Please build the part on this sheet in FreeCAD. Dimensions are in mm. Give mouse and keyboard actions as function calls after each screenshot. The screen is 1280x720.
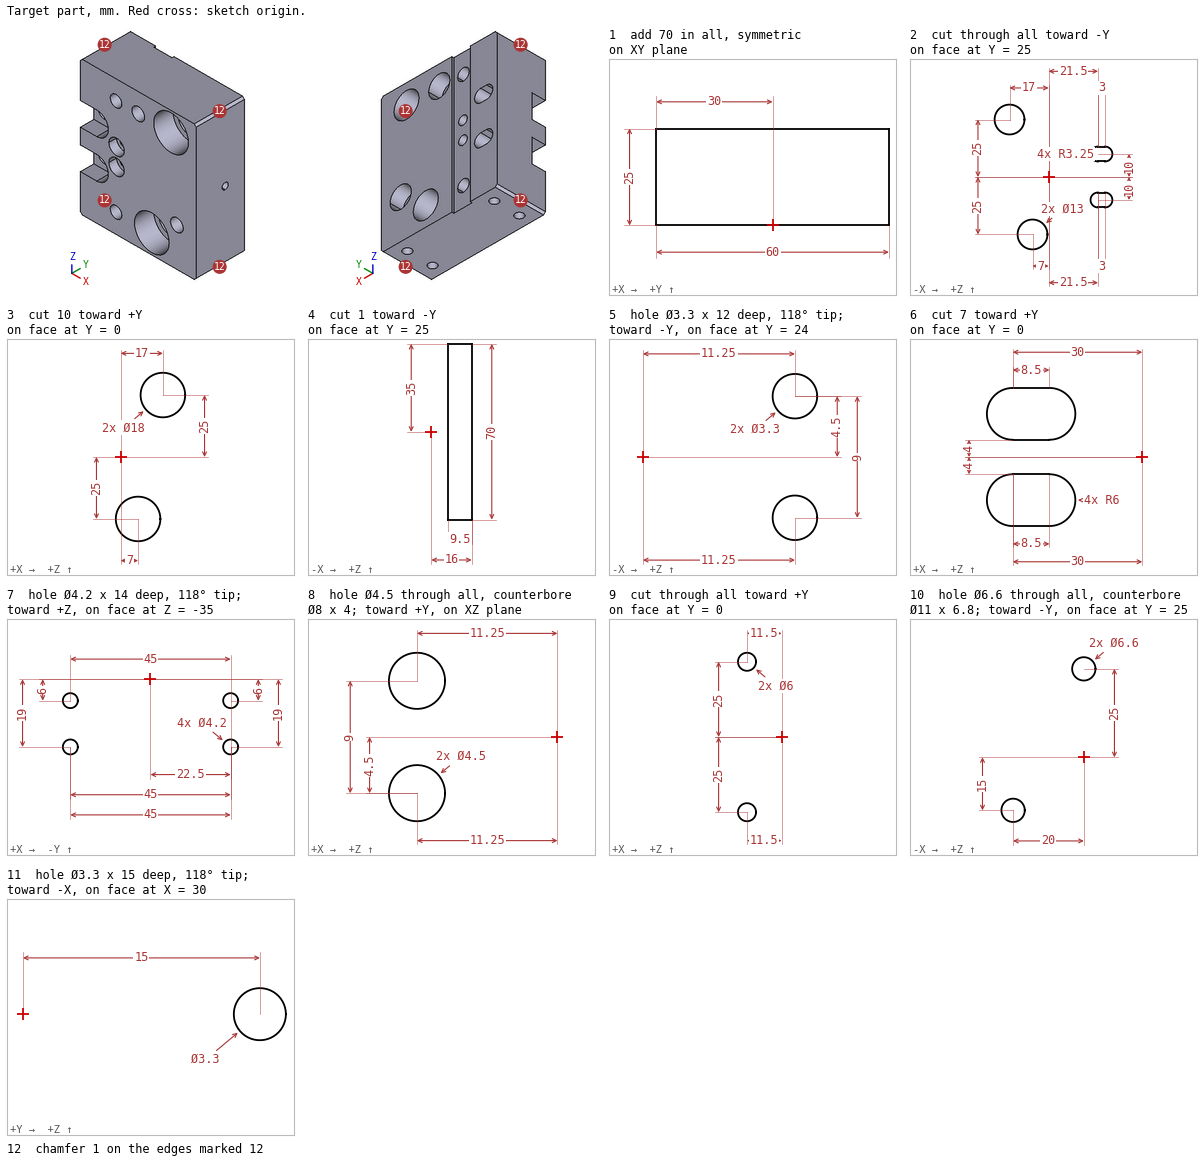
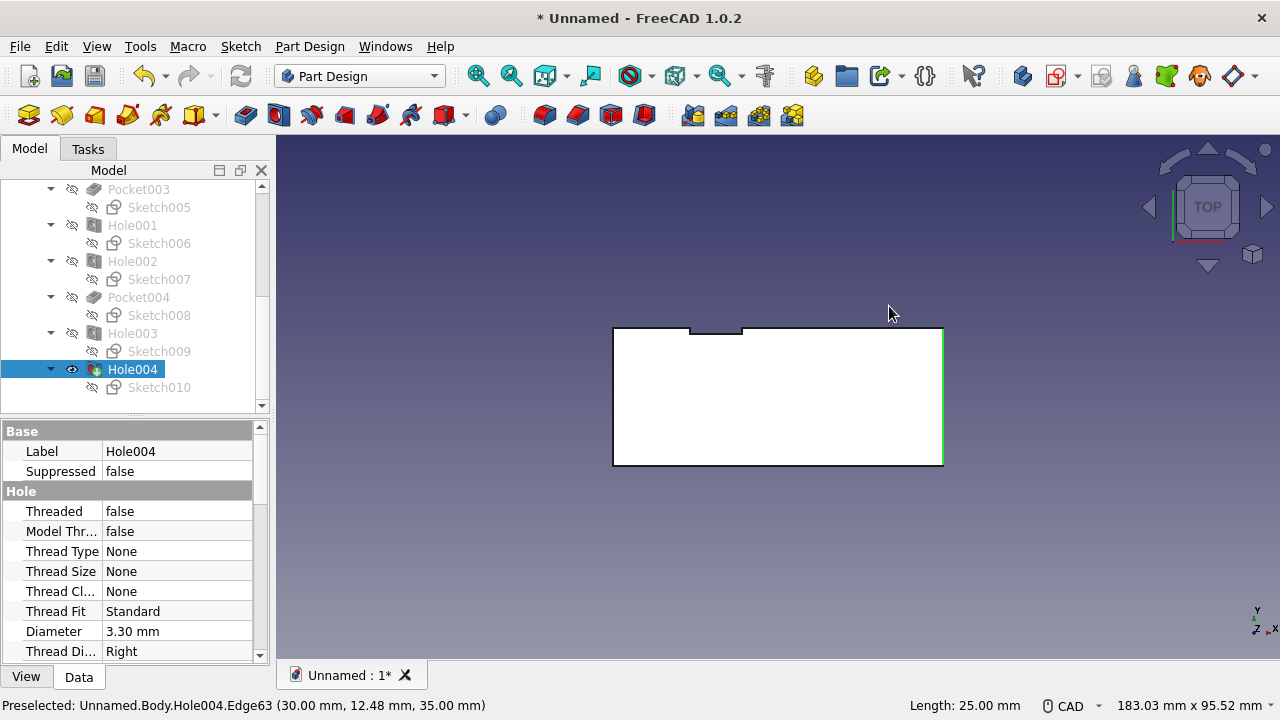
click(613, 396, ctrl)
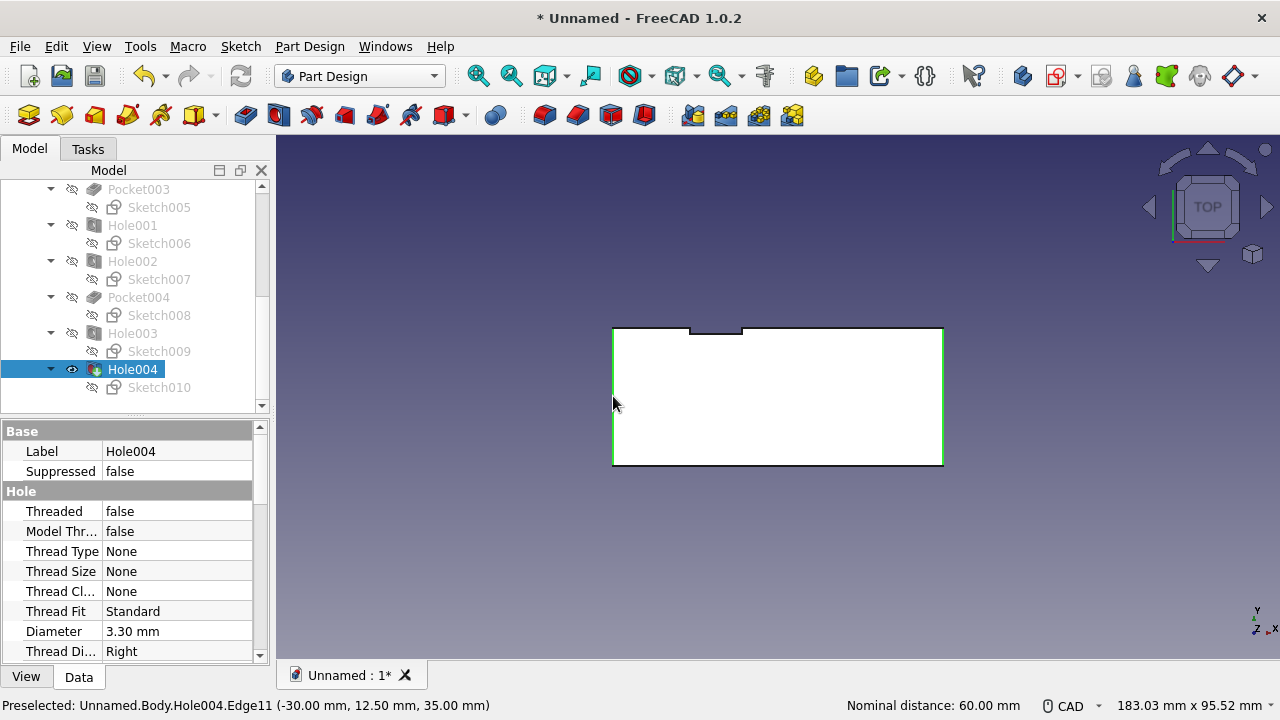
key(0)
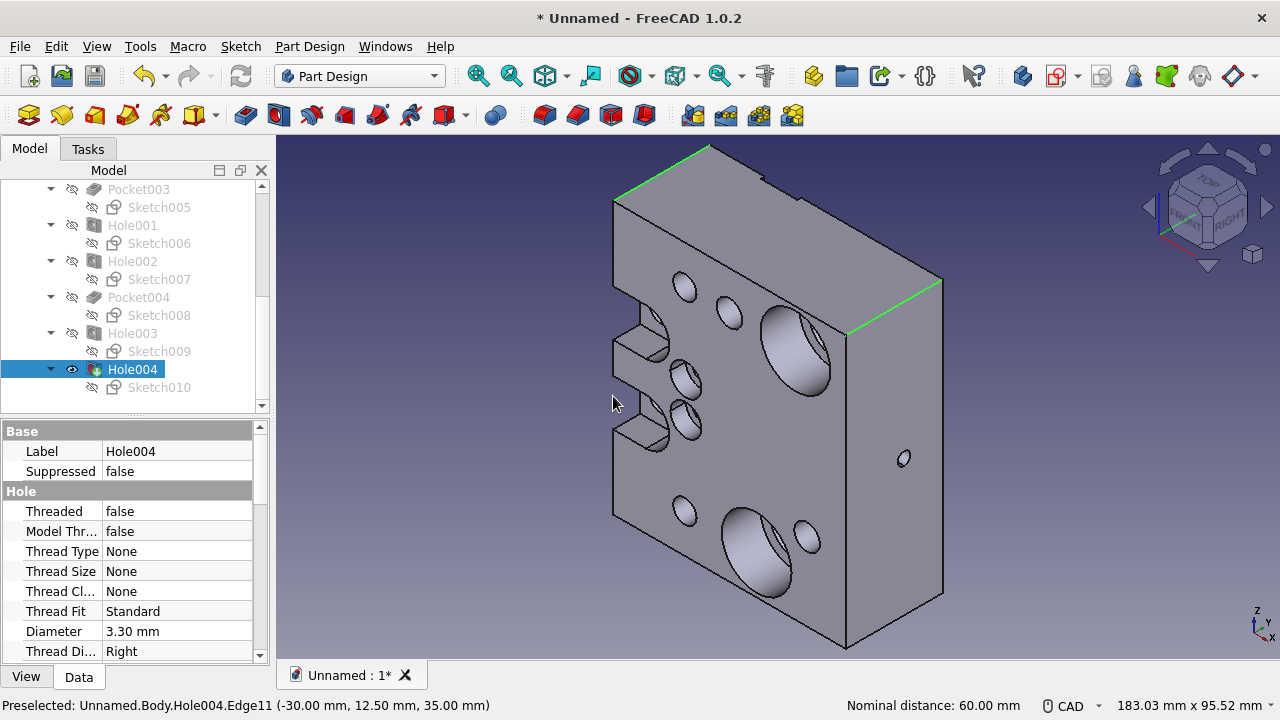
key(1)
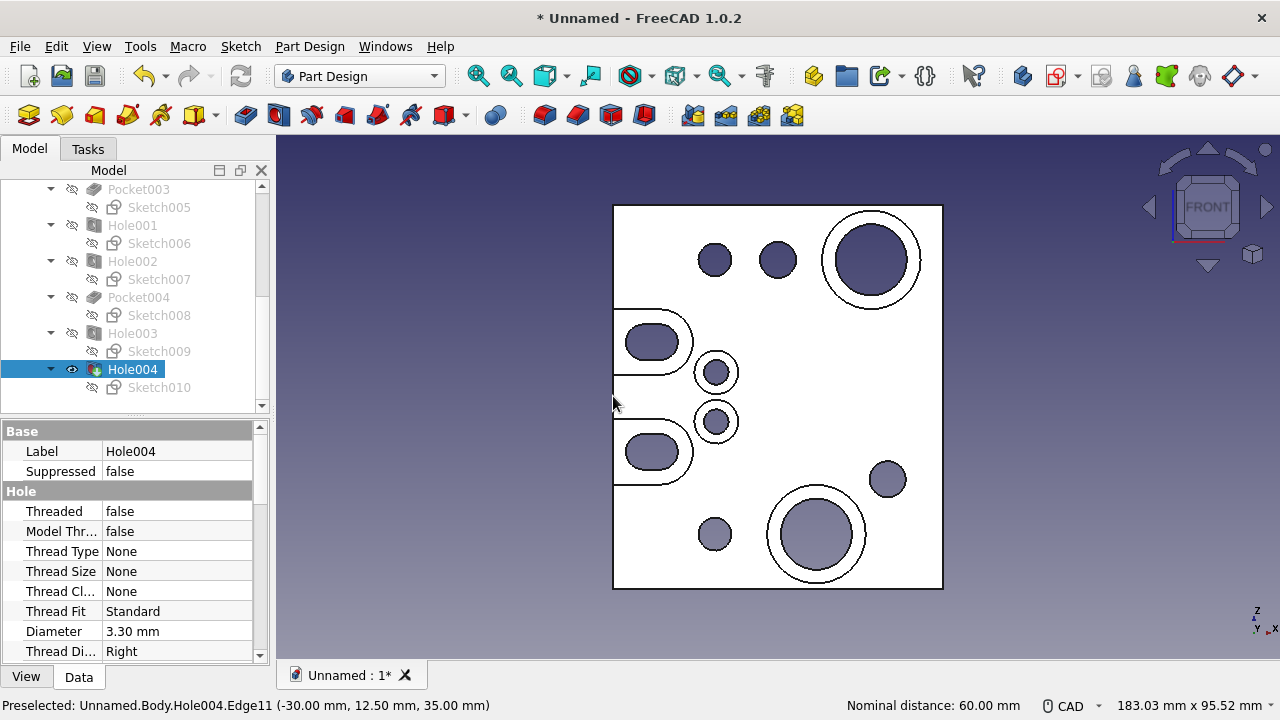
key(3)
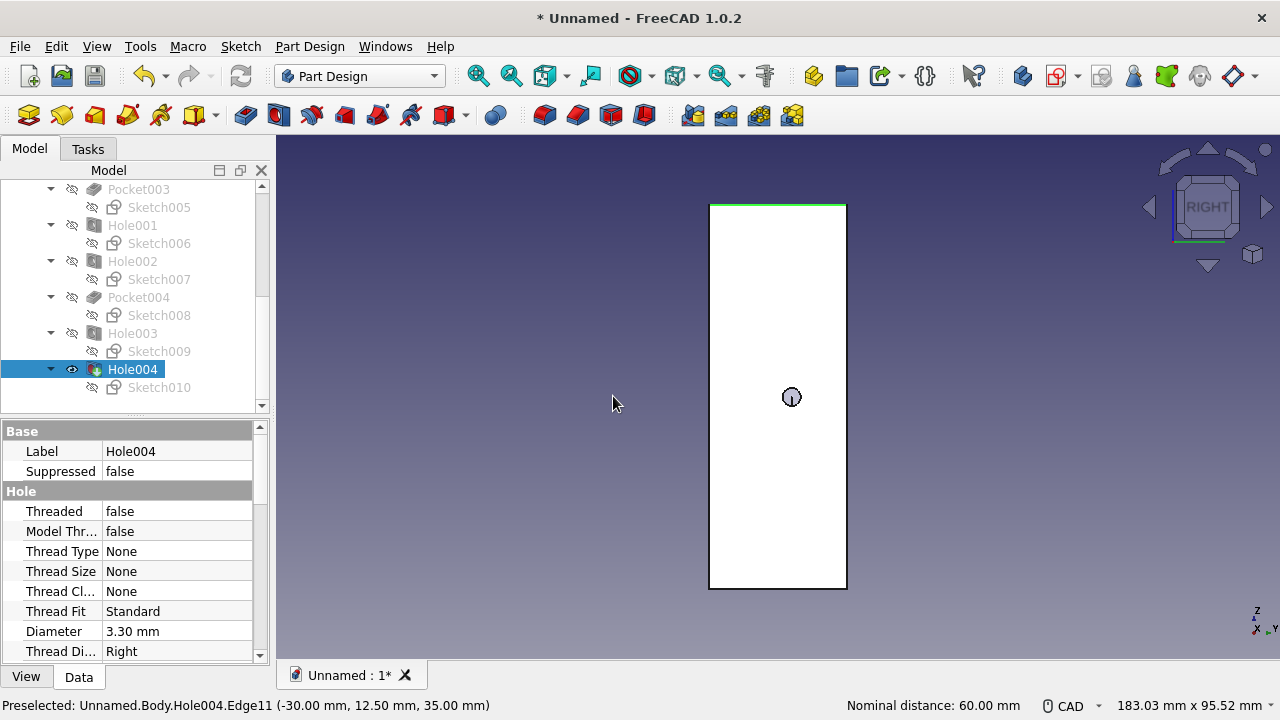
click(778, 588, ctrl)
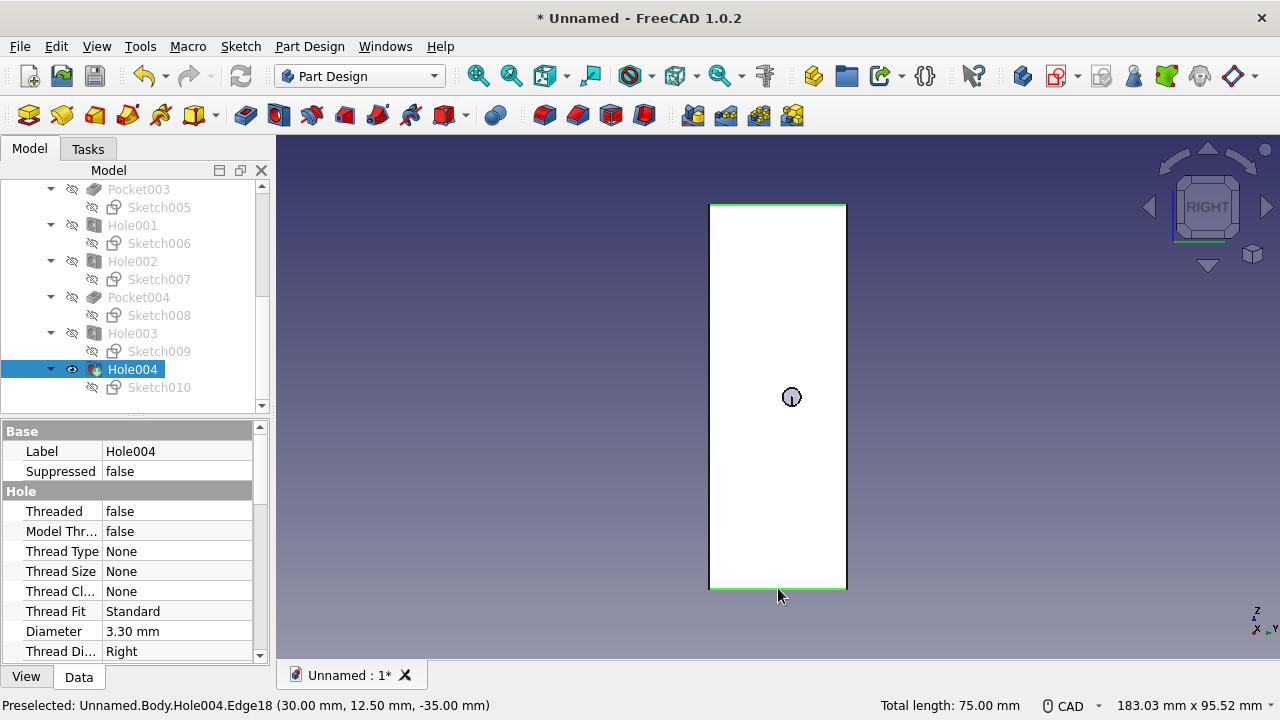
key(5)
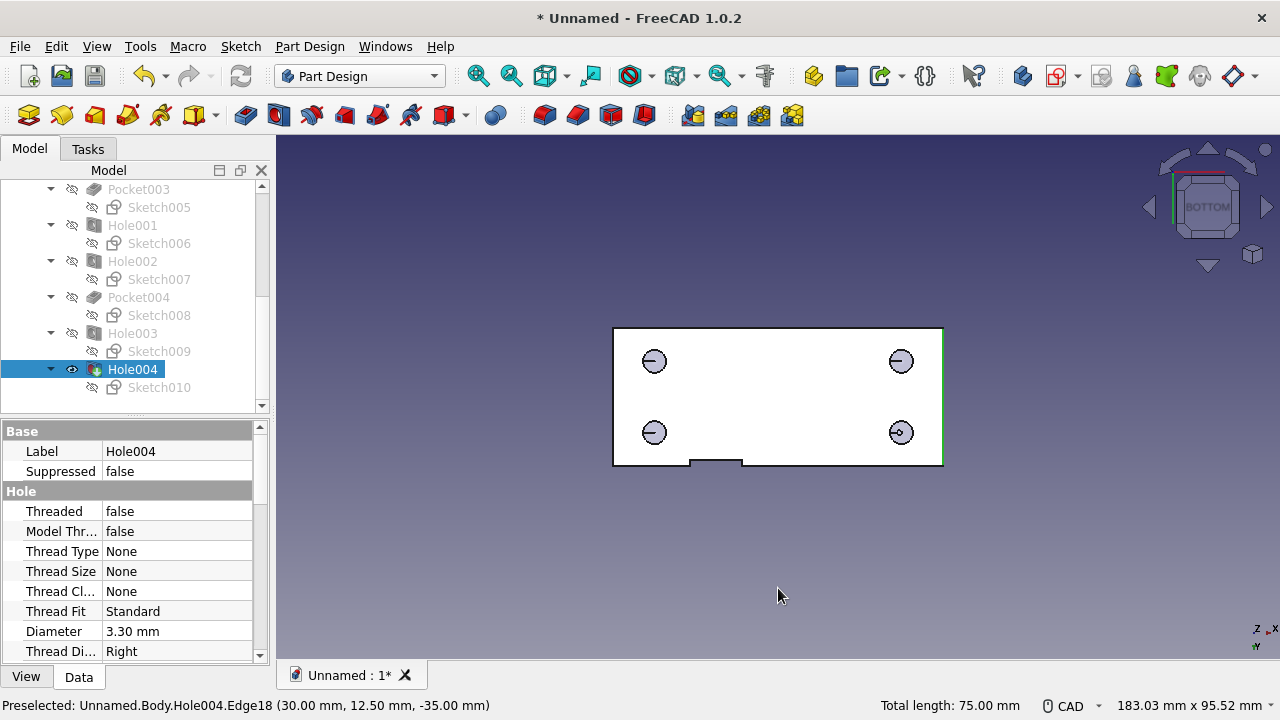
key(v)
key(f)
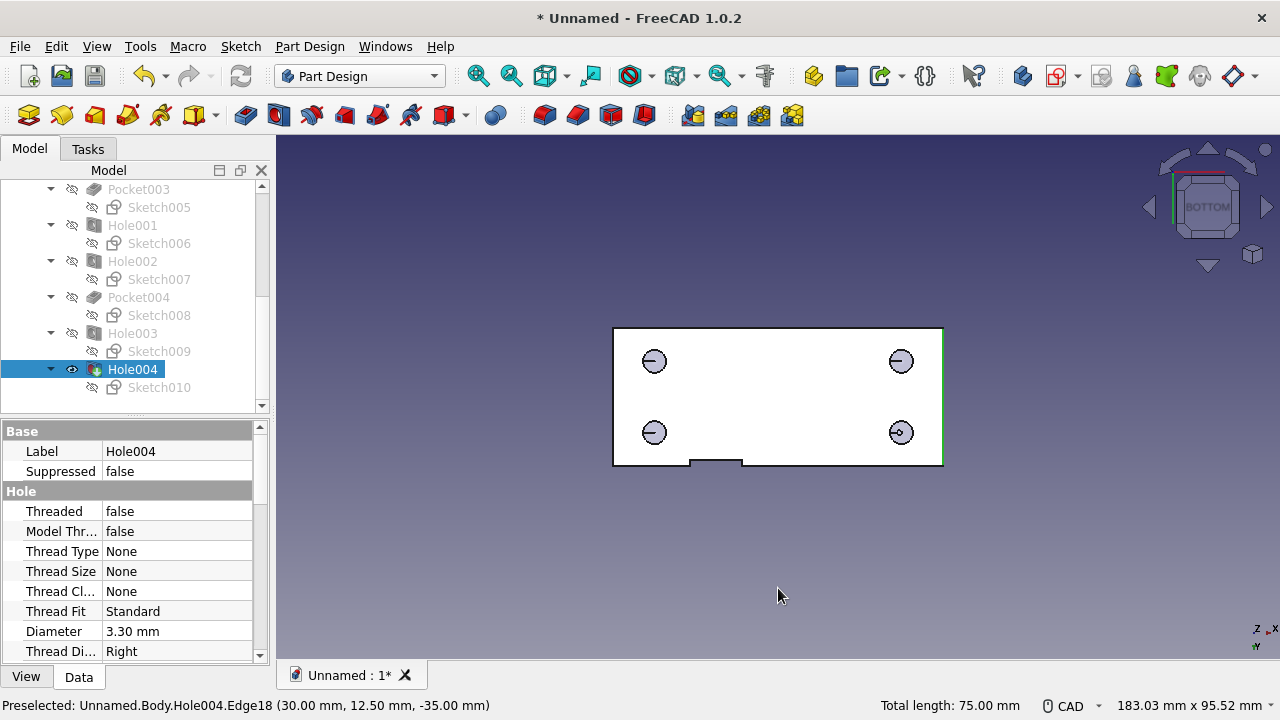
click(613, 396, ctrl)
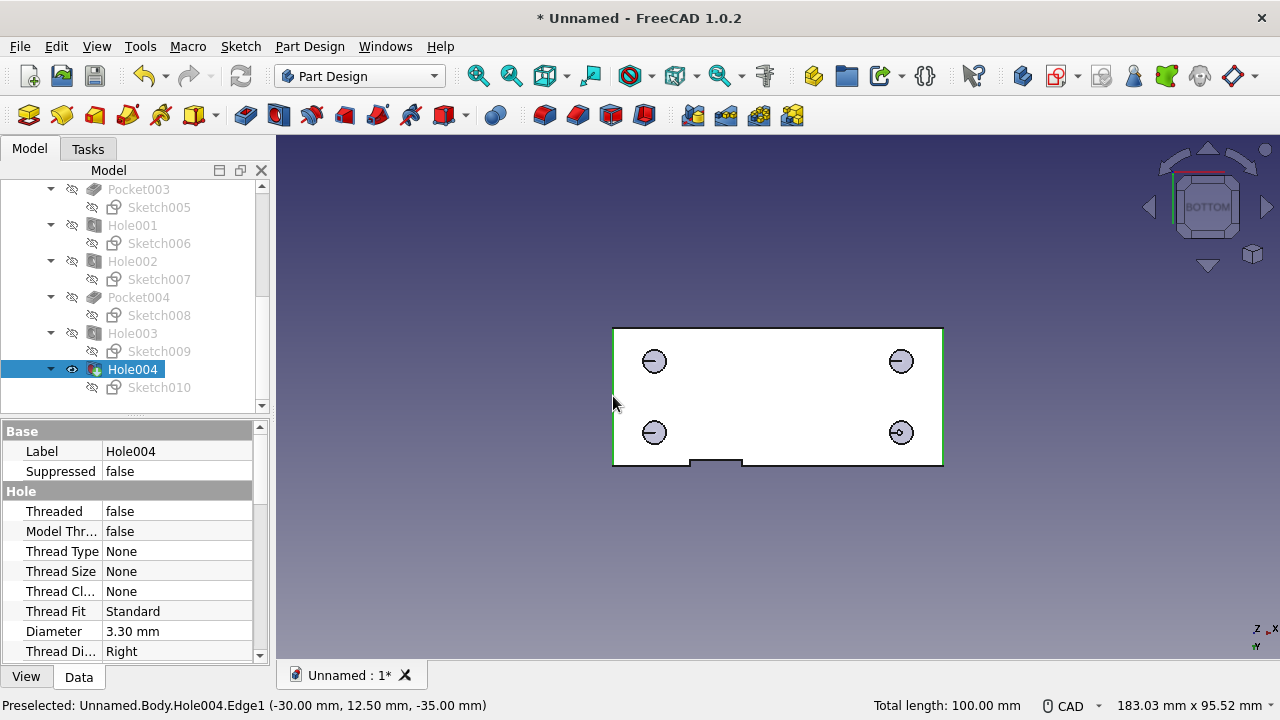
click(578, 116)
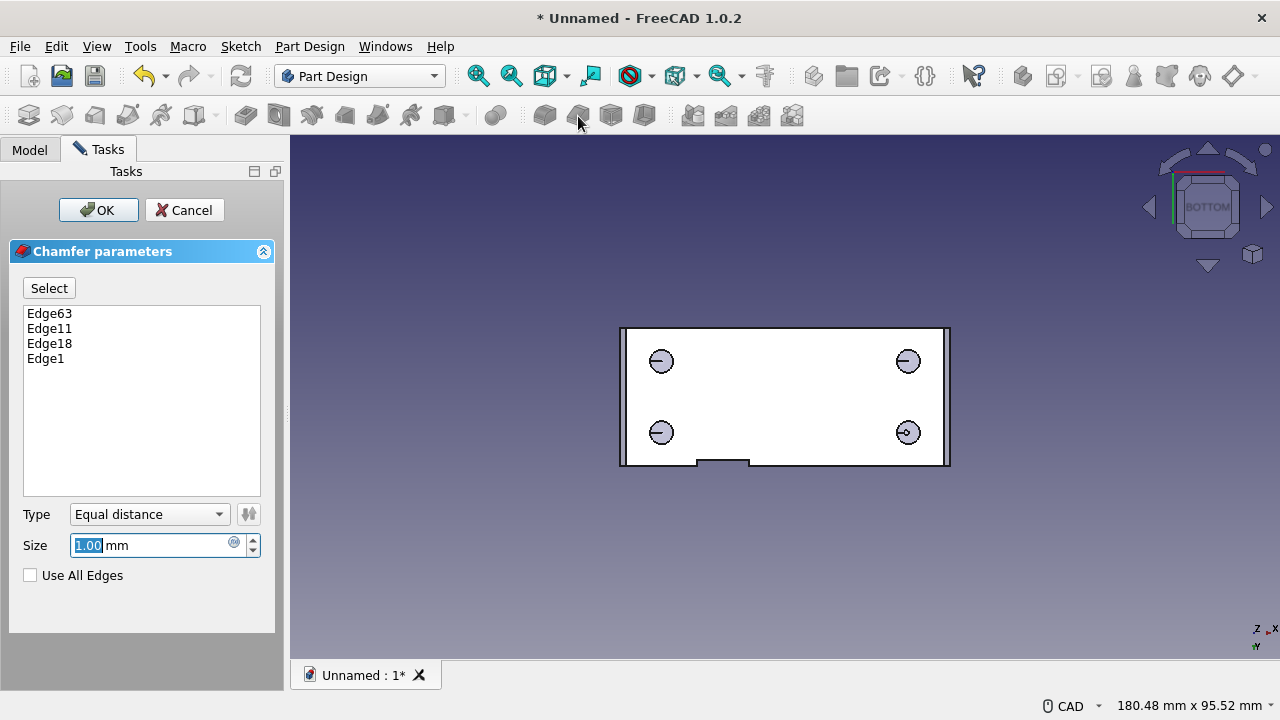
text(1)
key(Tab)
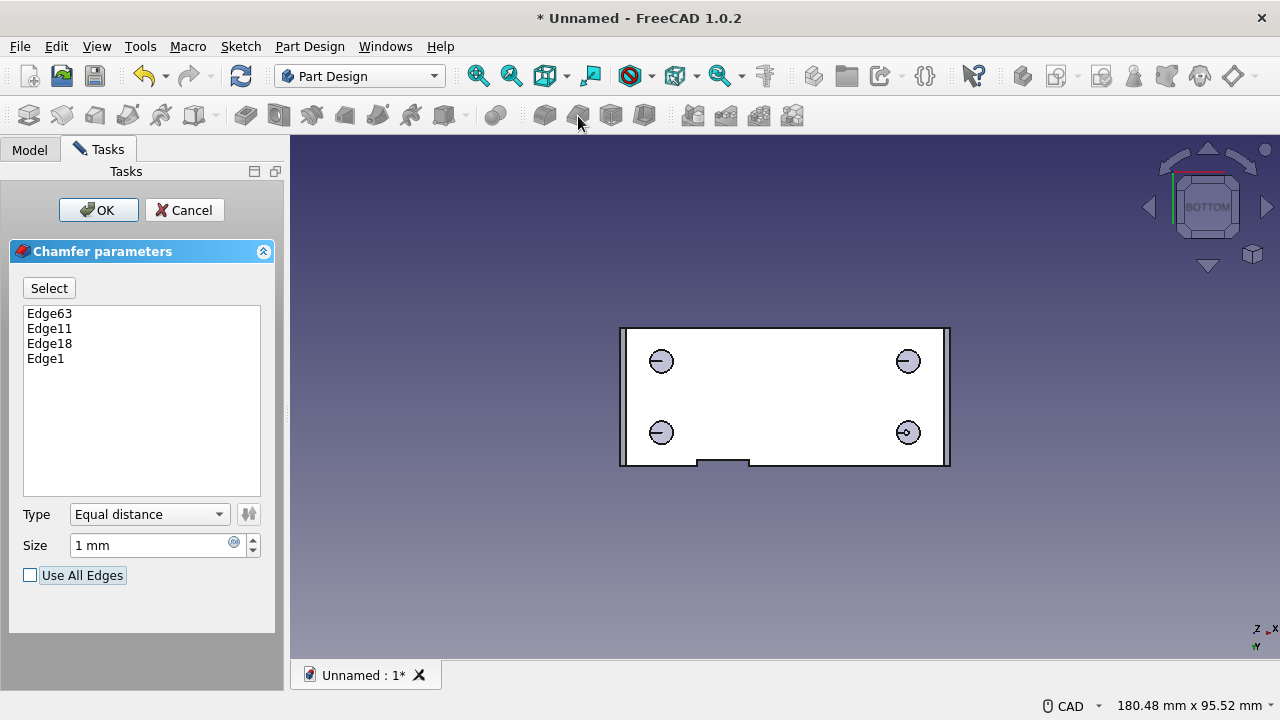
click(99, 210)